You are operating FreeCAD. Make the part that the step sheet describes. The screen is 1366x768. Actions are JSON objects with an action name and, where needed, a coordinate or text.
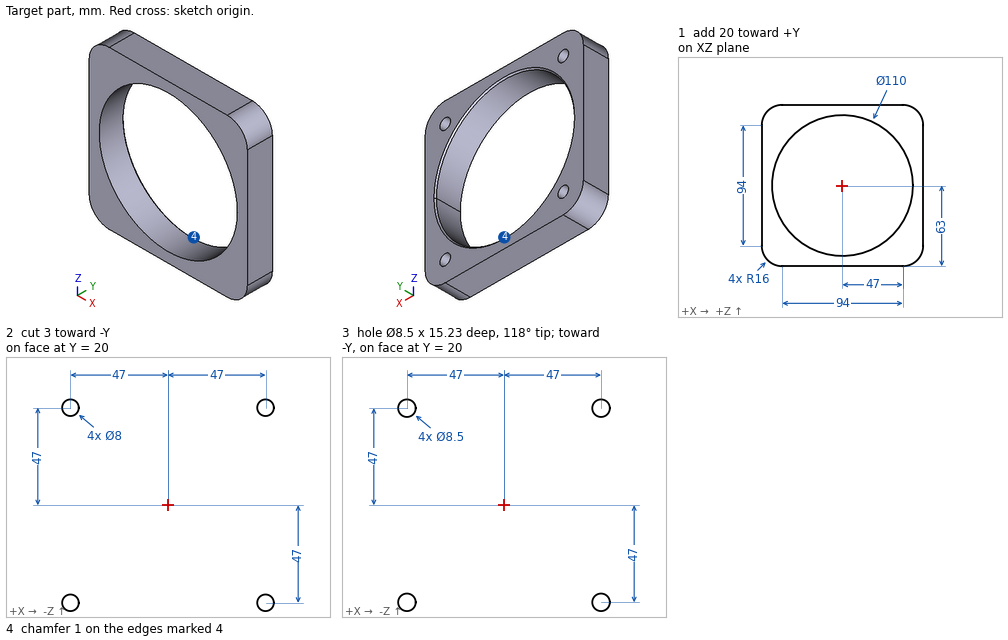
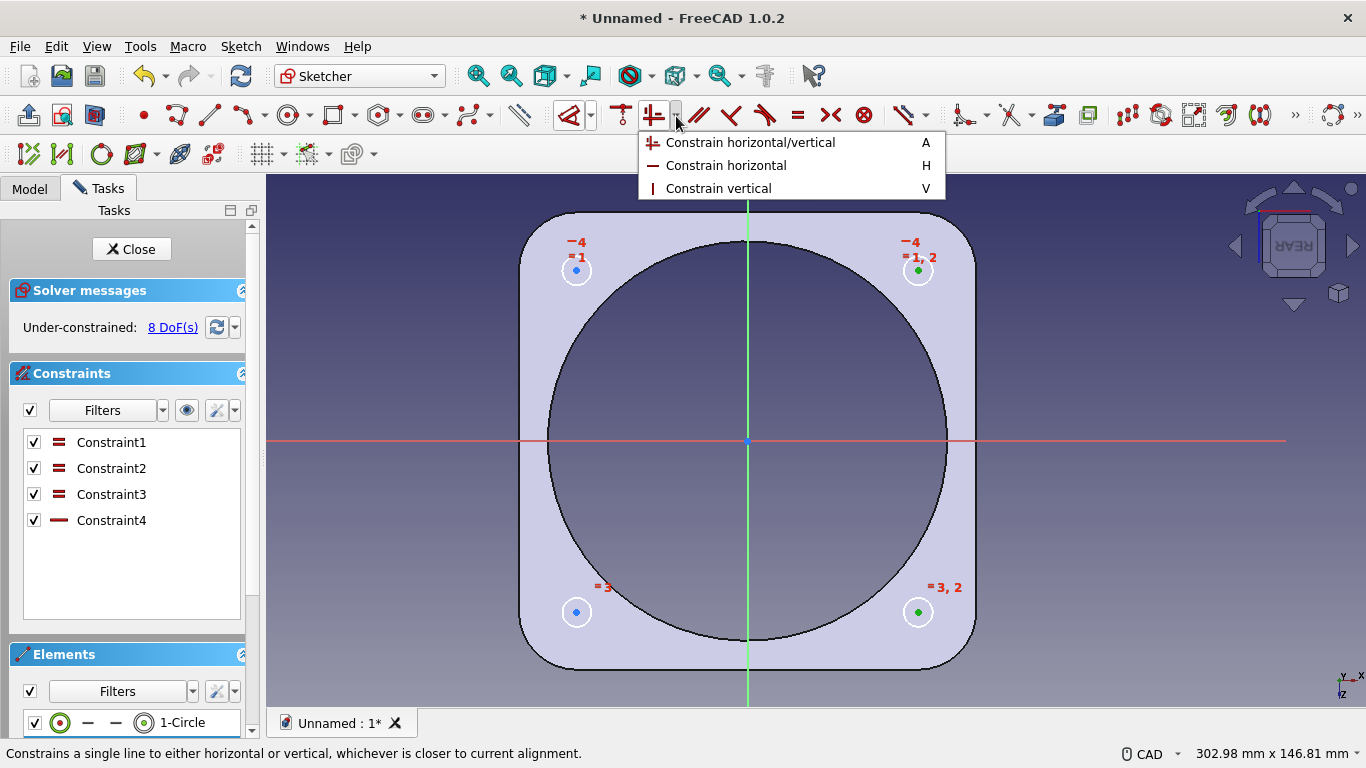
{"action": "left_click", "coordinate": [792, 188]}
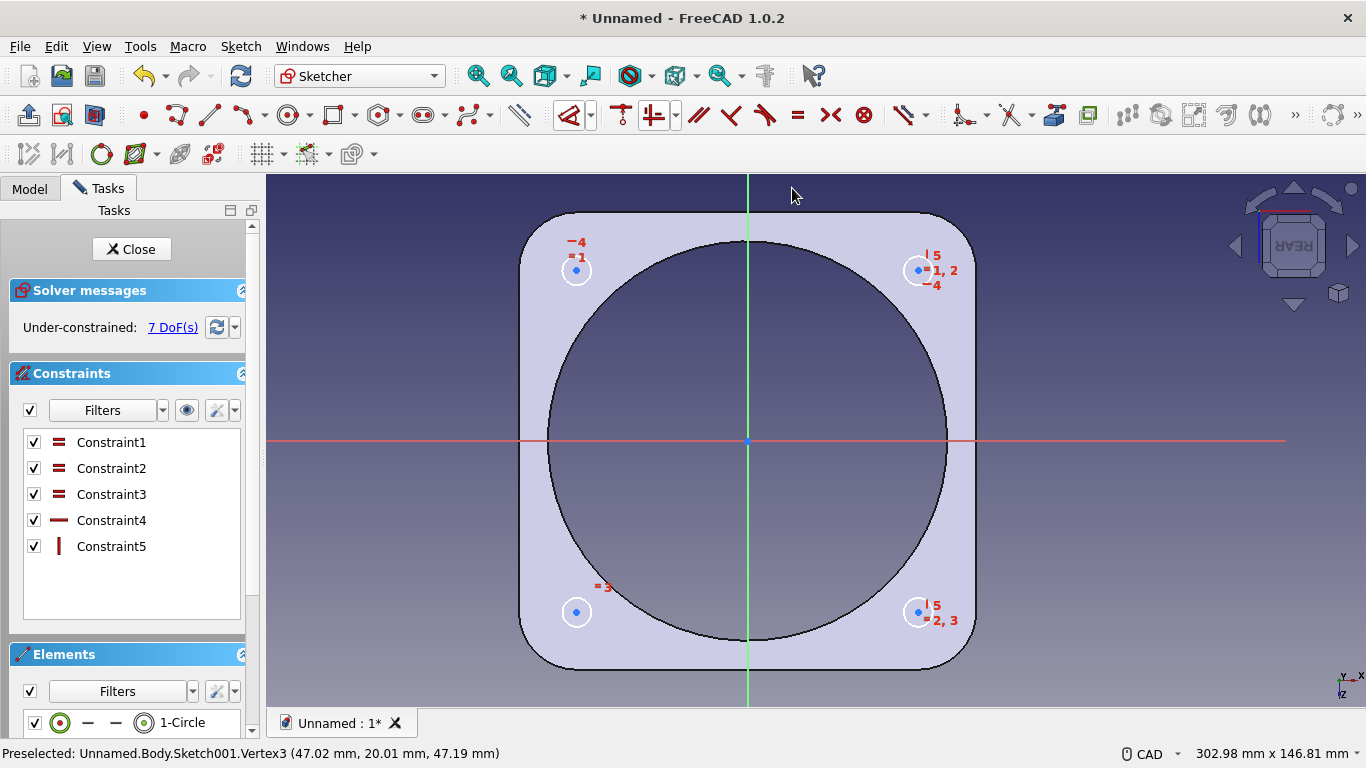
{"action": "left_click", "coordinate": [577, 271]}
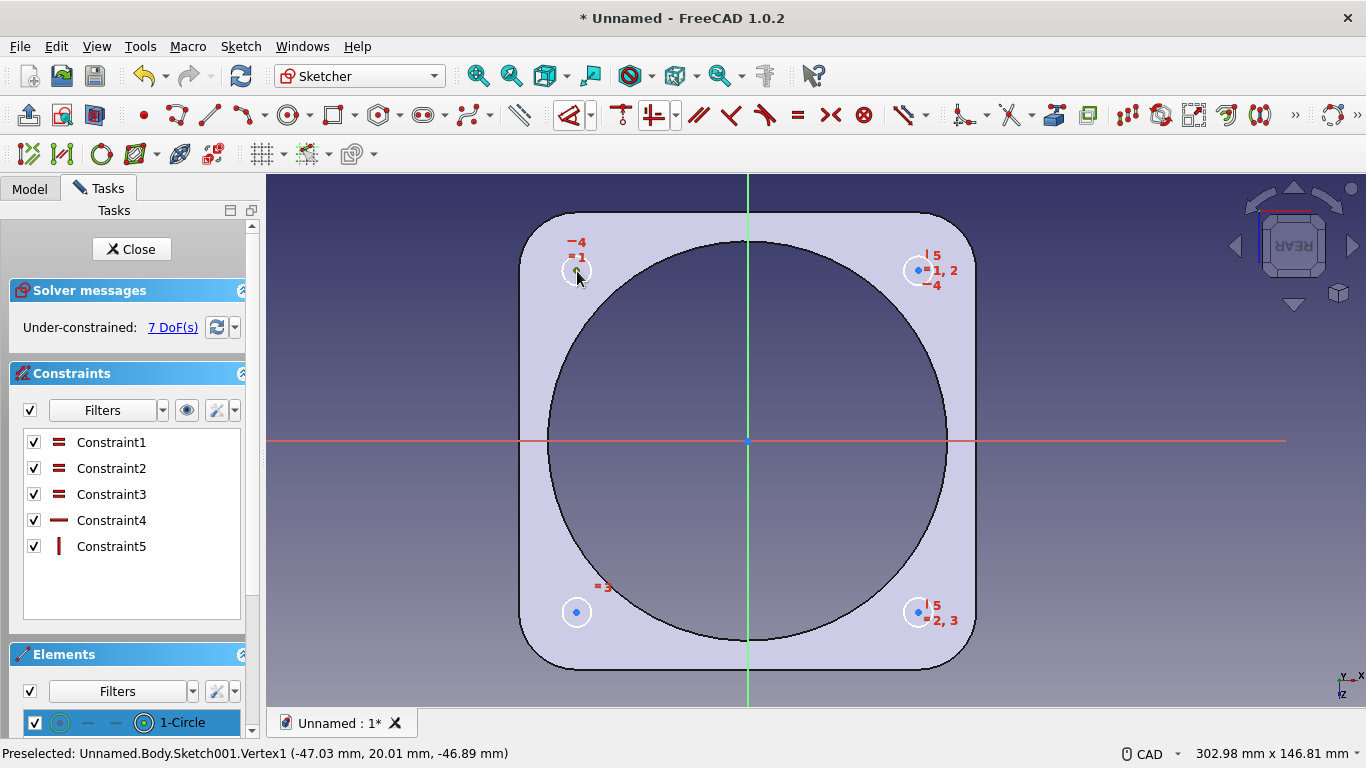
{"action": "left_click", "coordinate": [577, 612]}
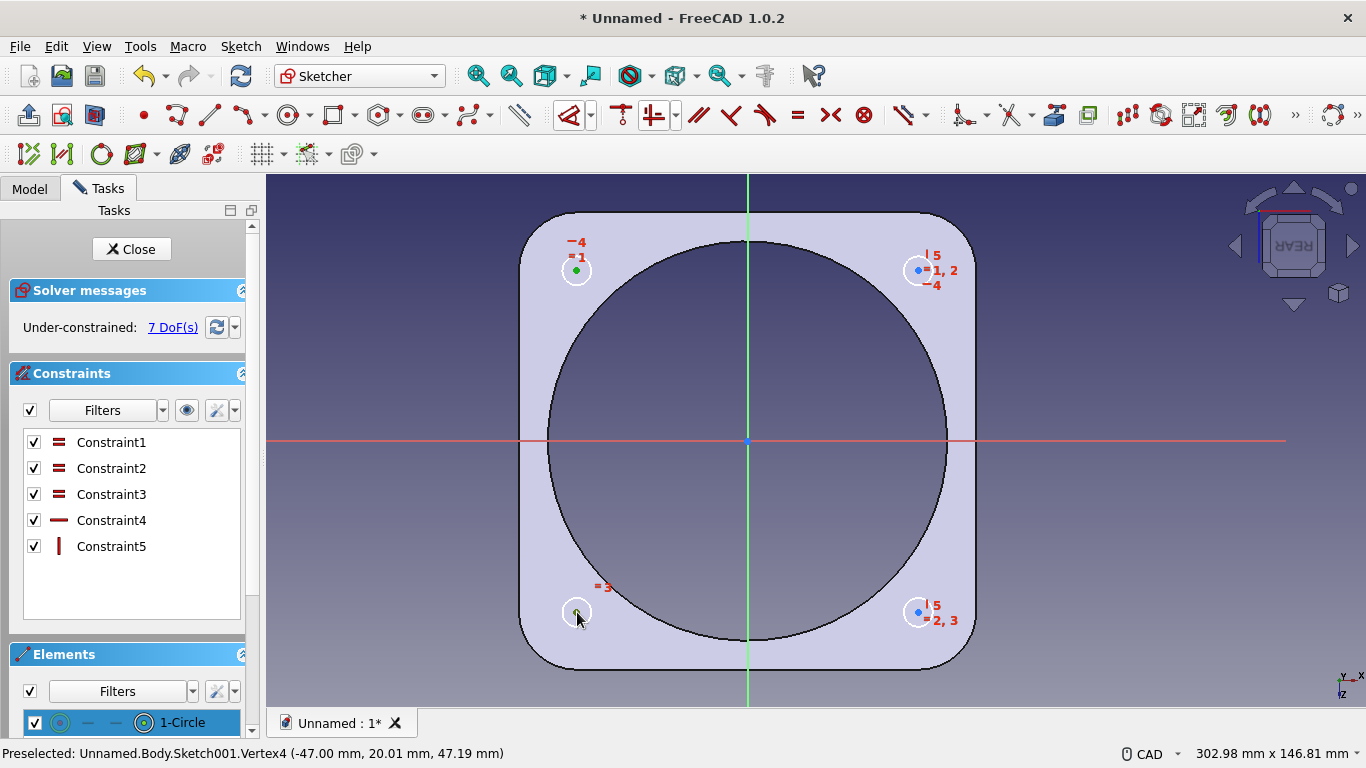
{"action": "key", "text": "v"}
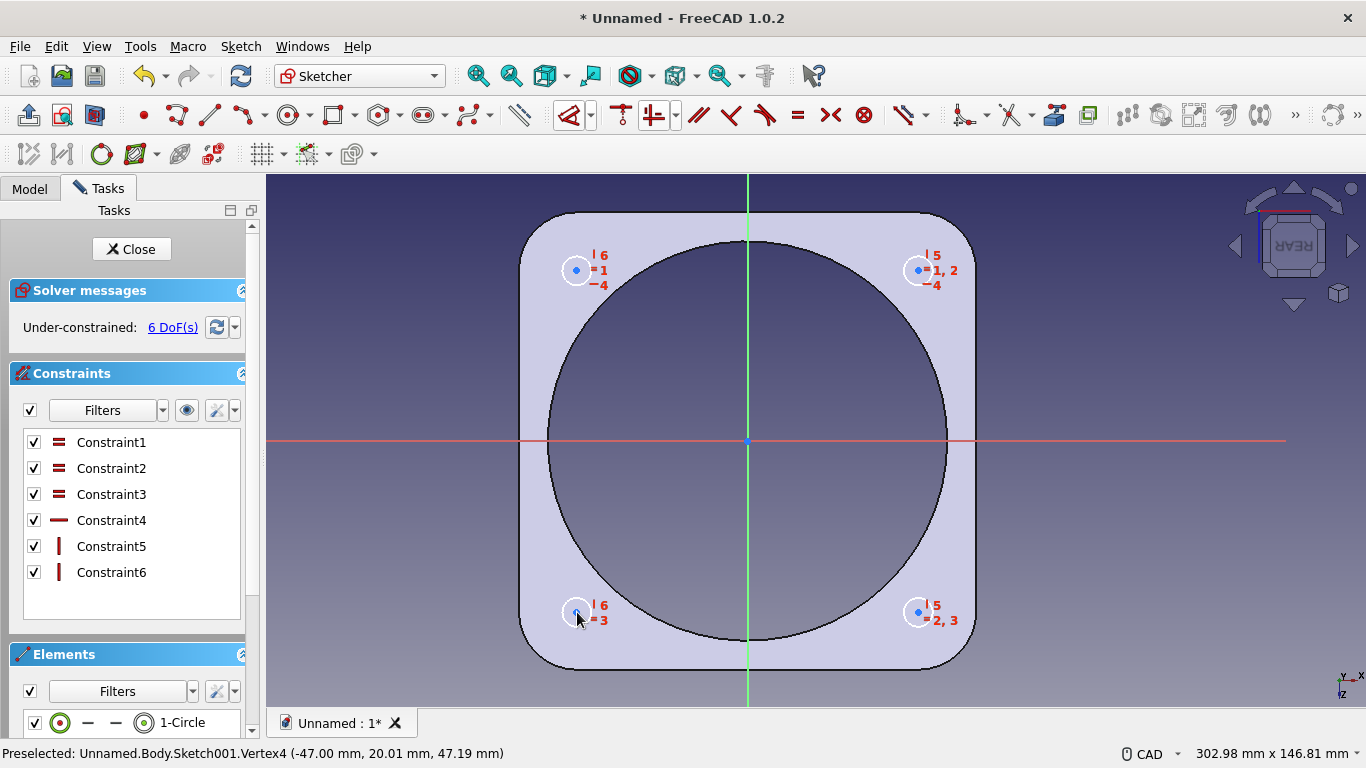
{"action": "left_click", "coordinate": [918, 612]}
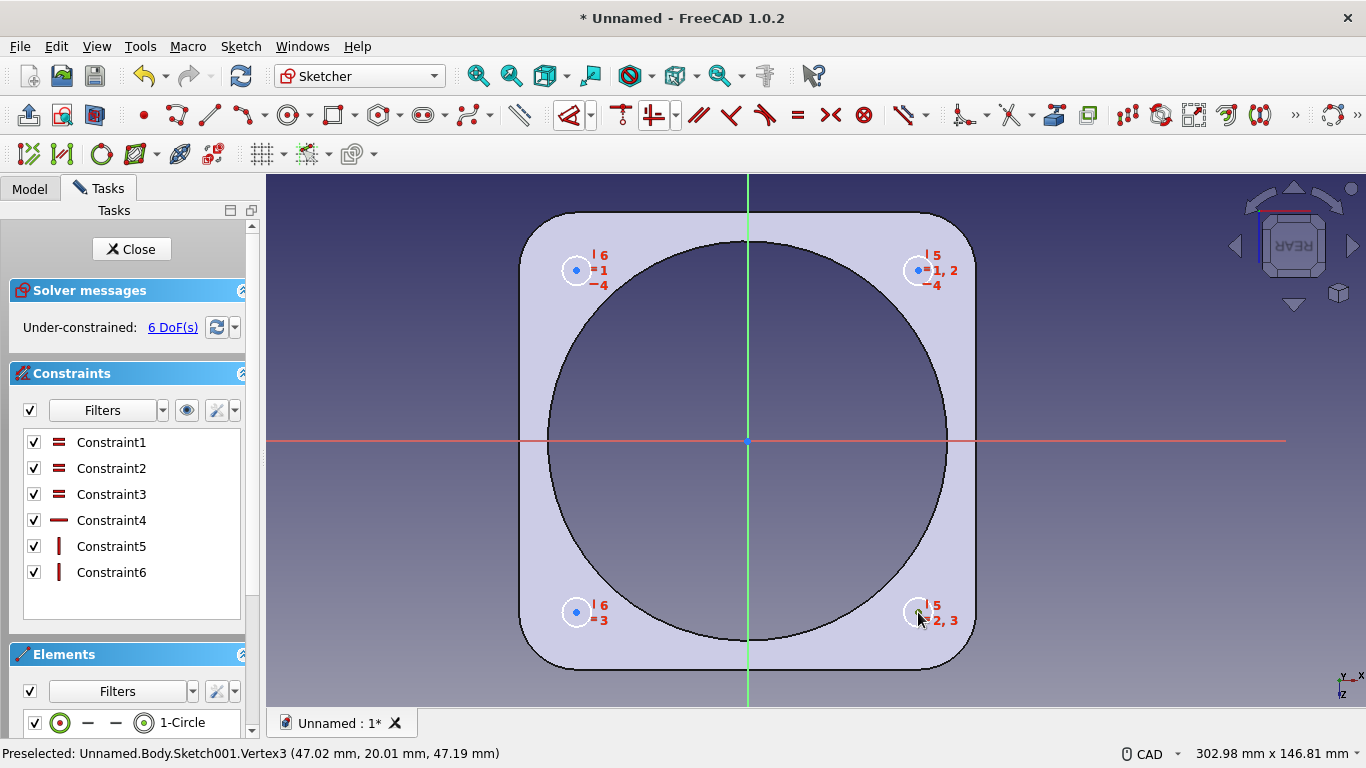
{"action": "left_click", "coordinate": [577, 612]}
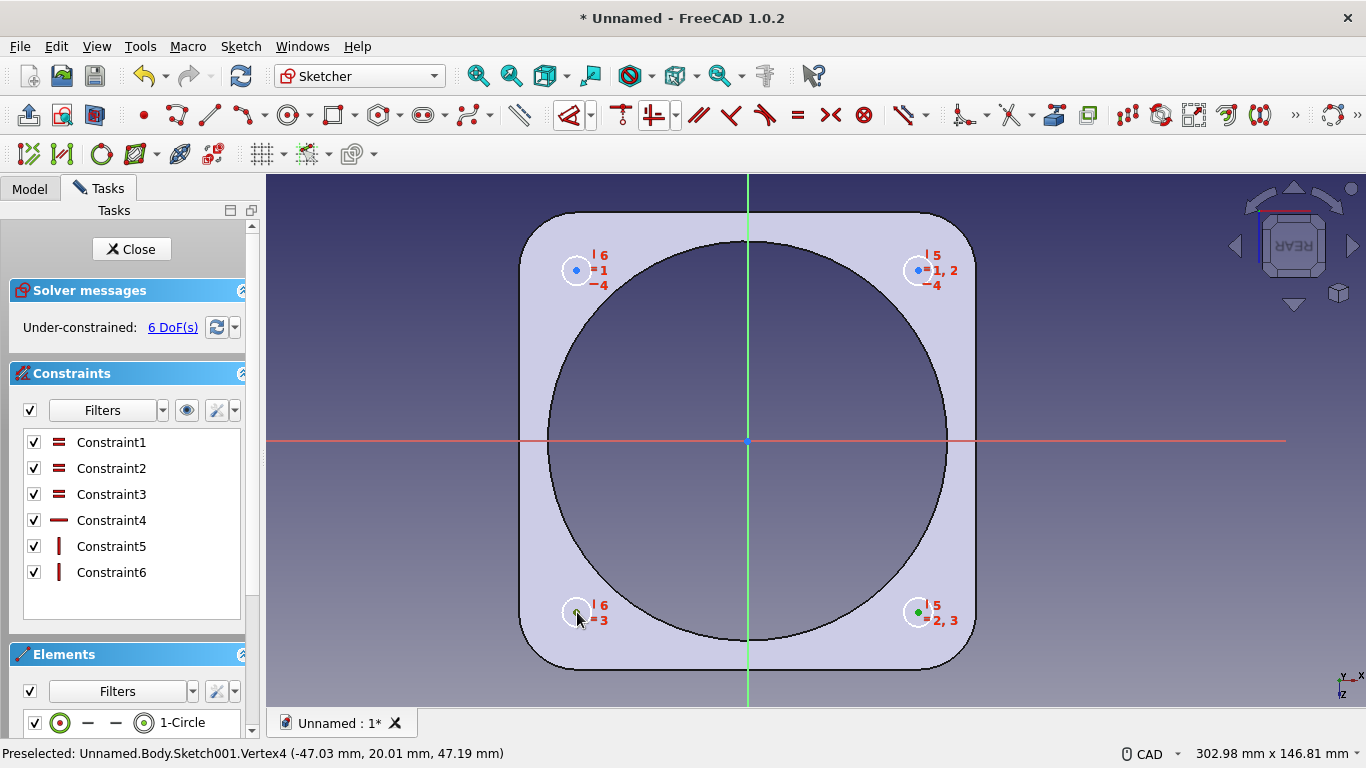
{"action": "left_click", "coordinate": [676, 116]}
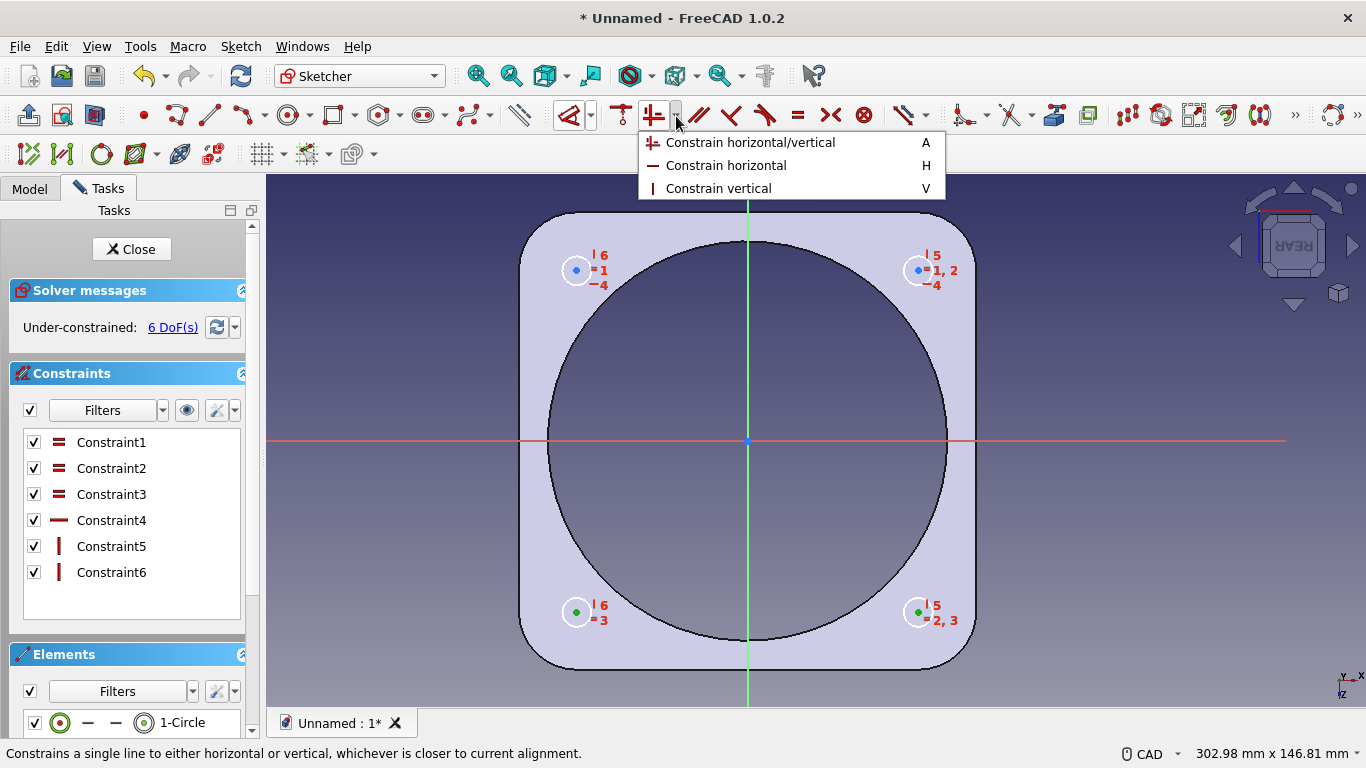
{"action": "left_click", "coordinate": [792, 166]}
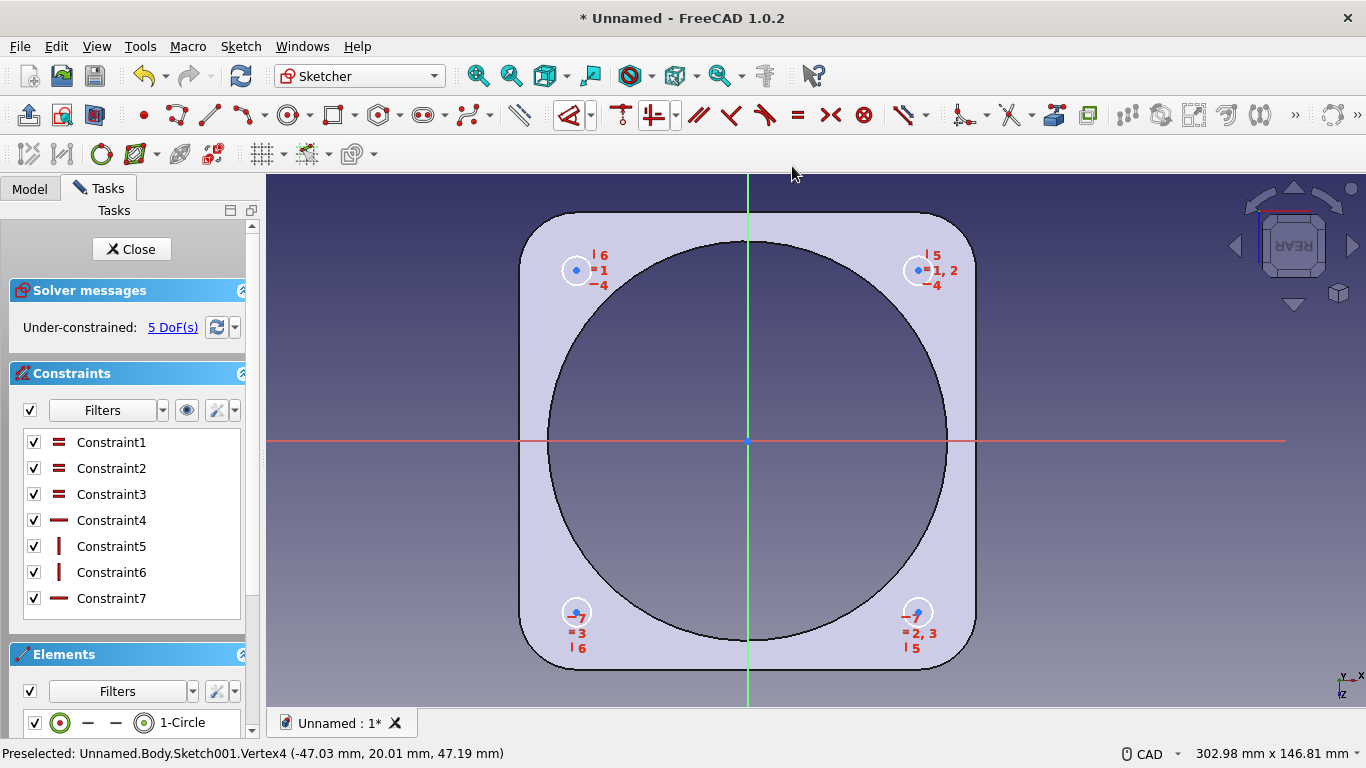
{"action": "scroll", "coordinate": [587, 261], "scroll_direction": "up", "scroll_amount": 2}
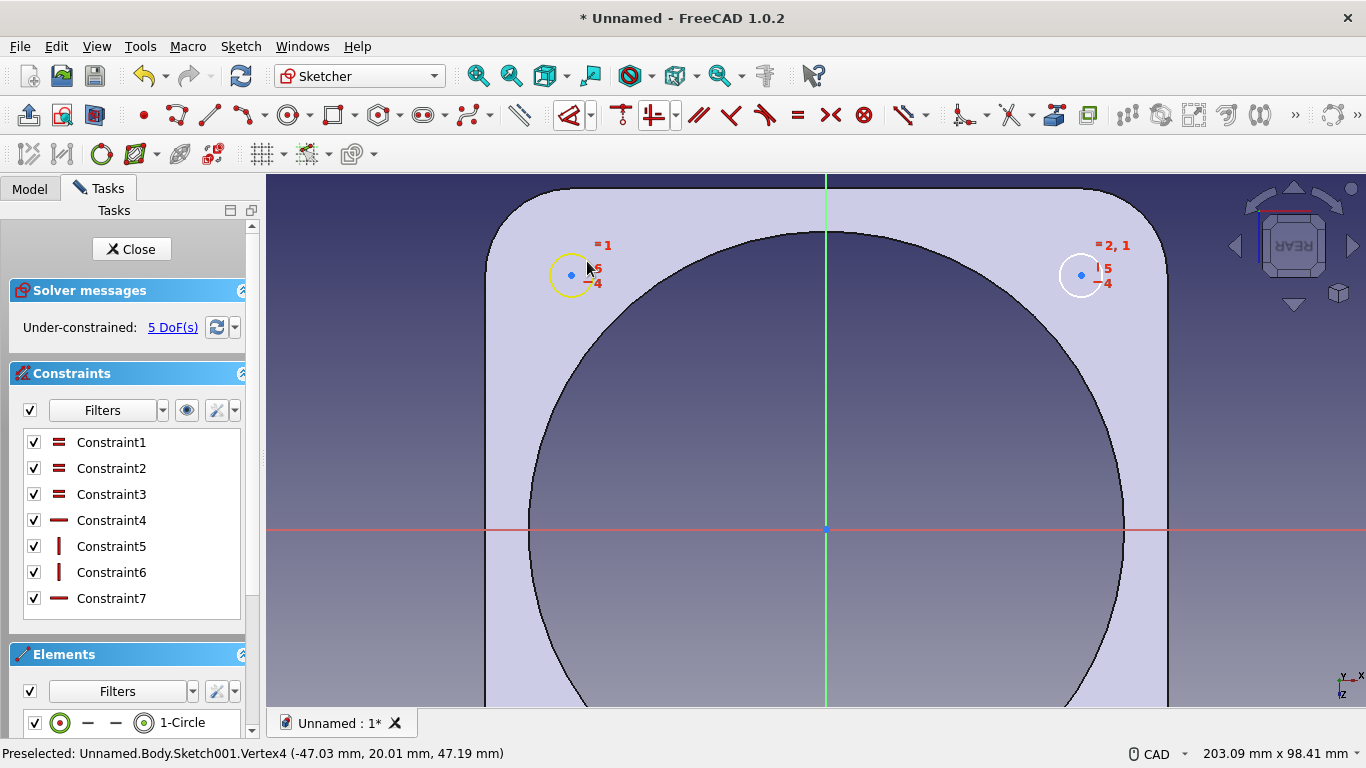
{"action": "left_click", "coordinate": [556, 260]}